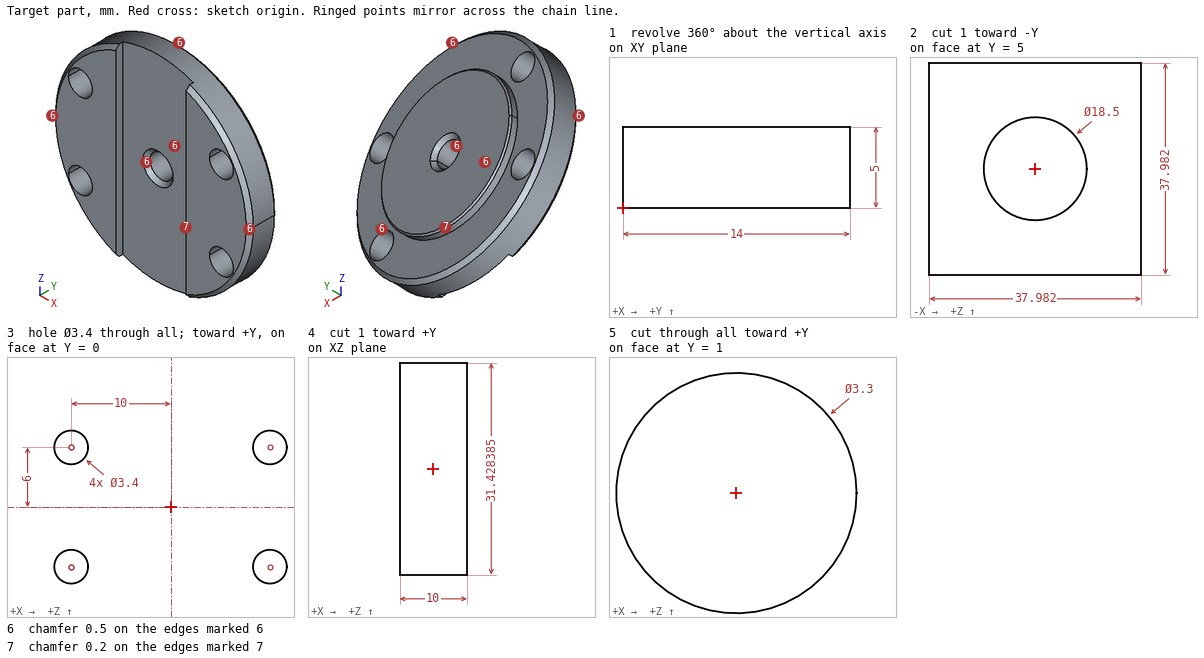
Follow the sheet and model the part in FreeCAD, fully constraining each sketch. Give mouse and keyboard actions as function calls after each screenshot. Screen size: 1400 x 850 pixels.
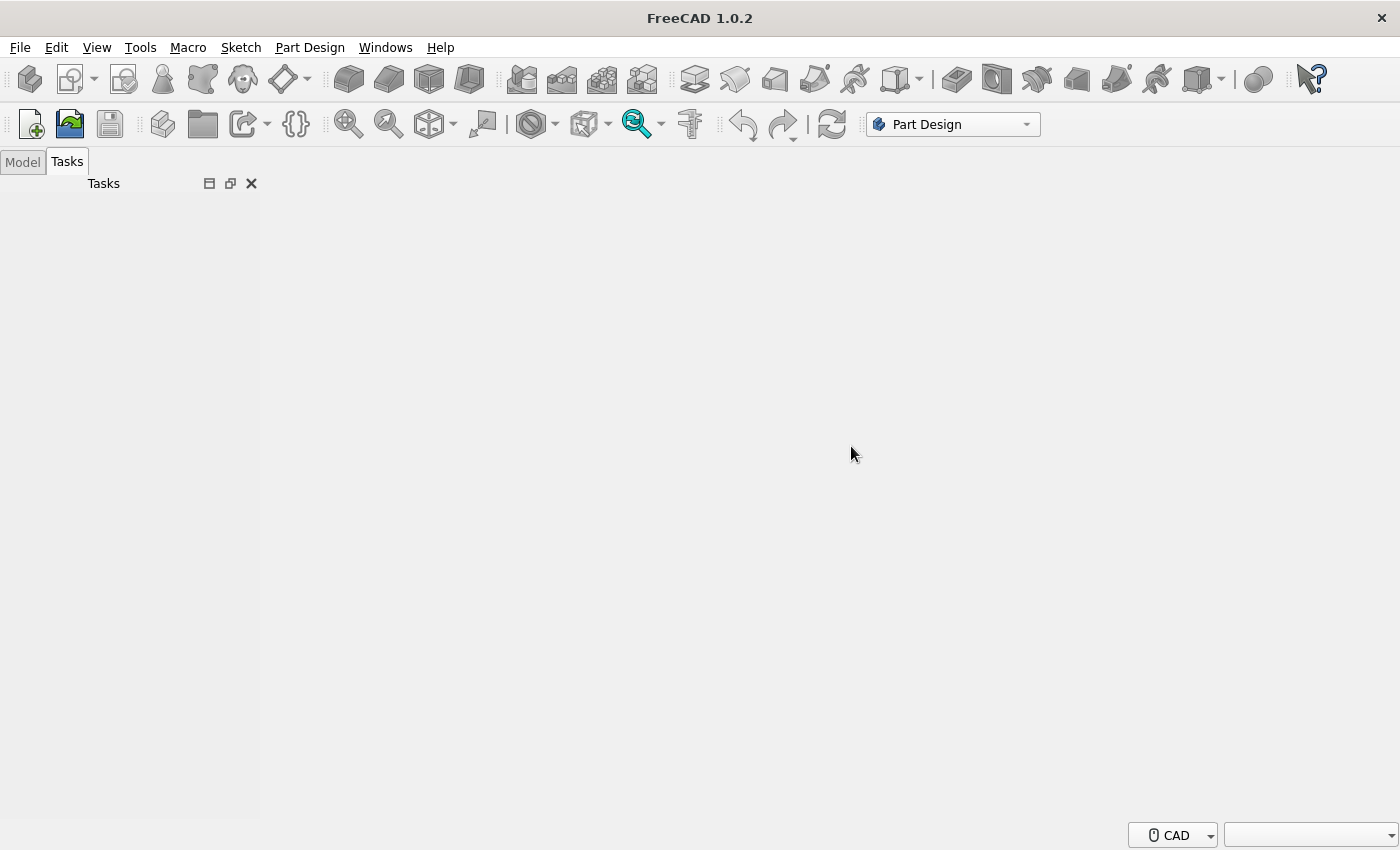
key(ctrl+n)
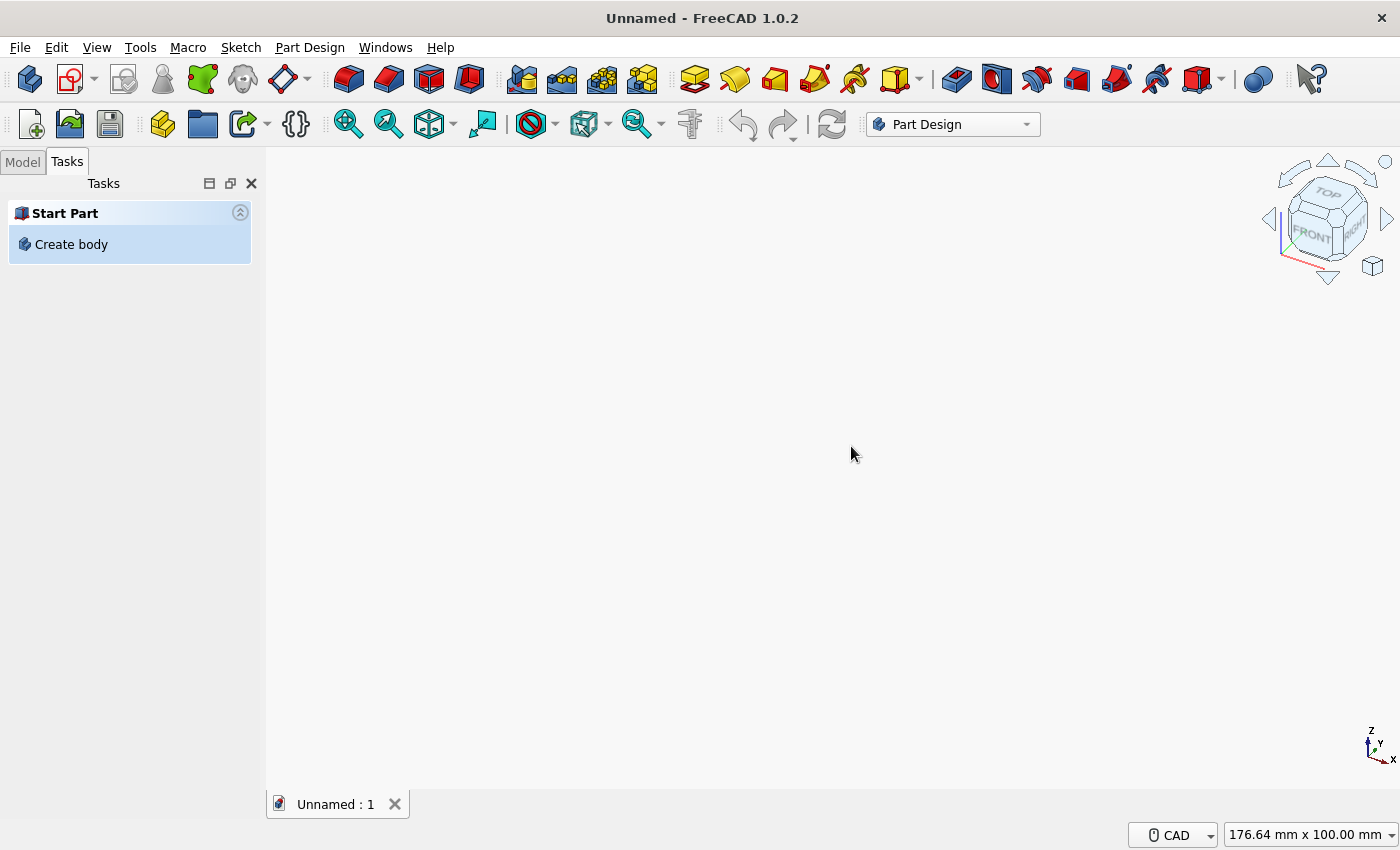
click(70, 80)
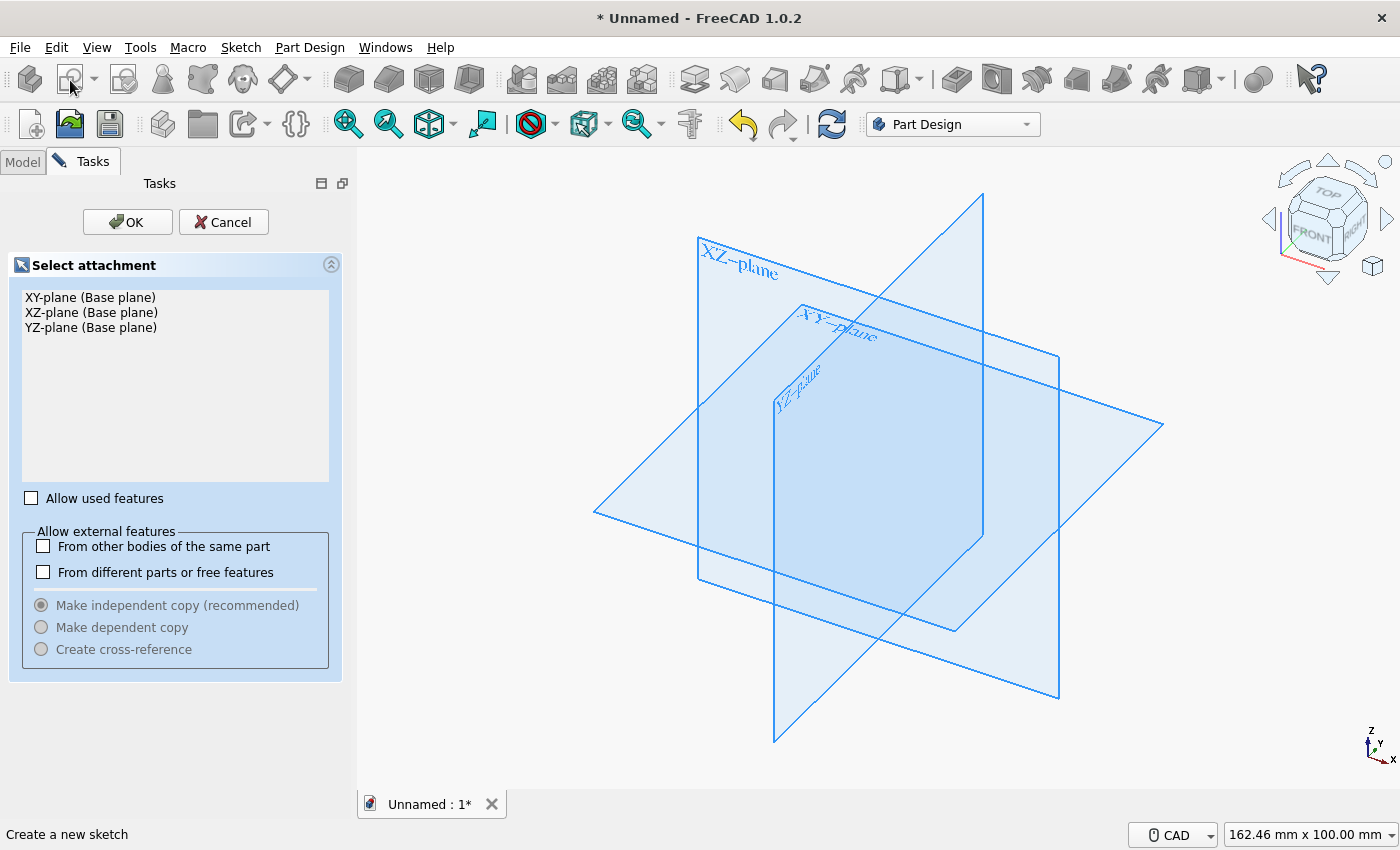
click(82, 298)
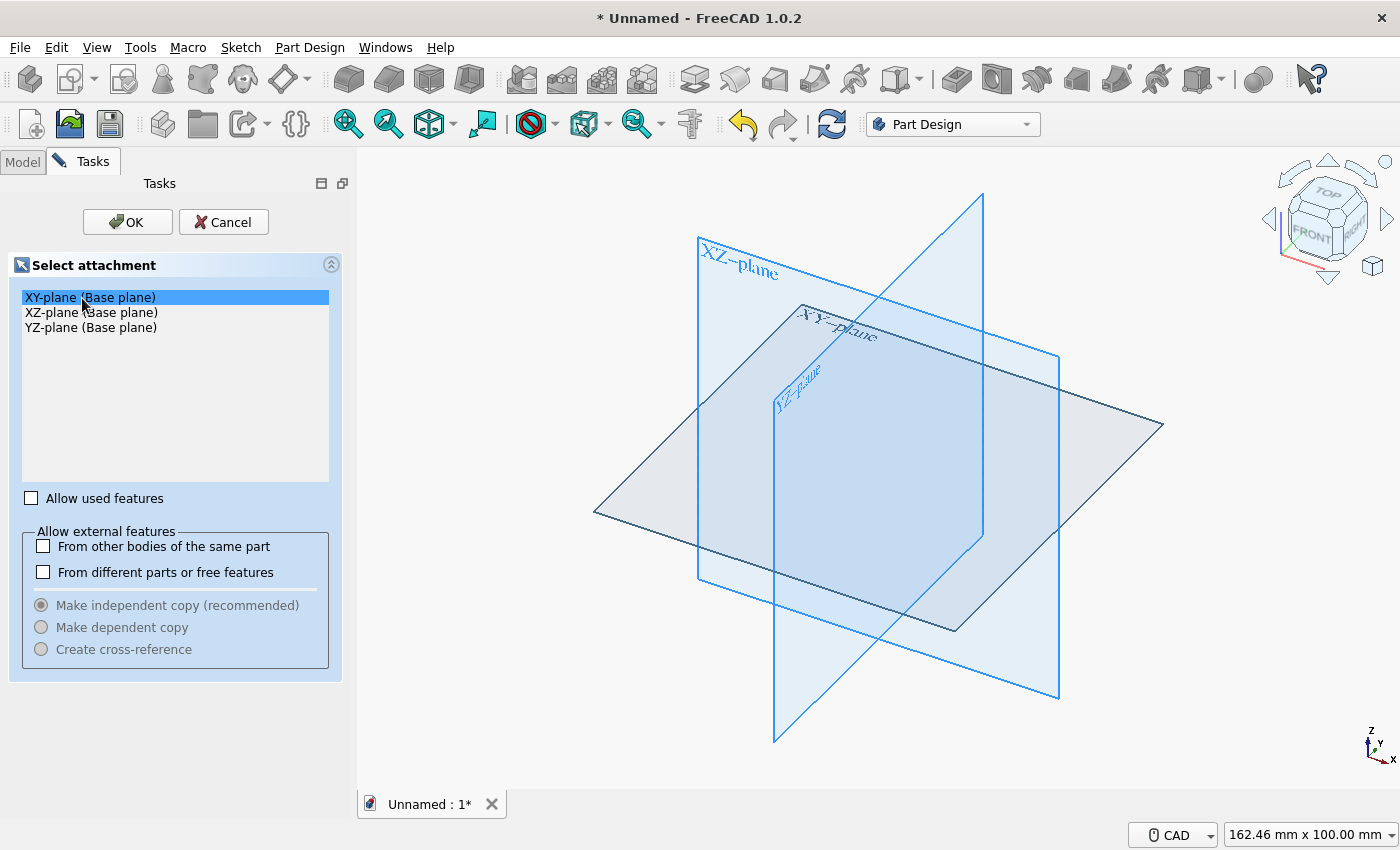
click(128, 222)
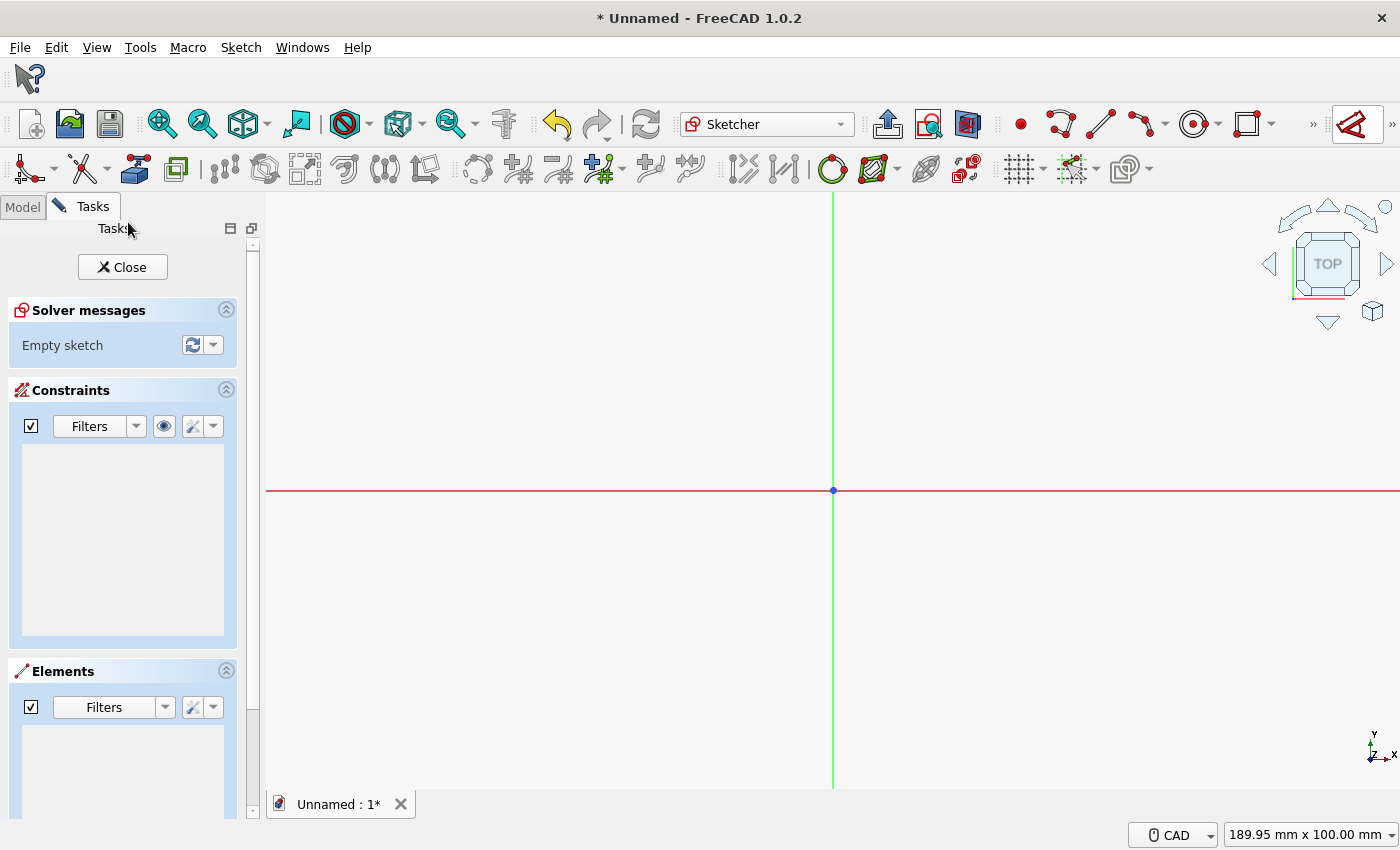
scroll(892, 473, up, 10)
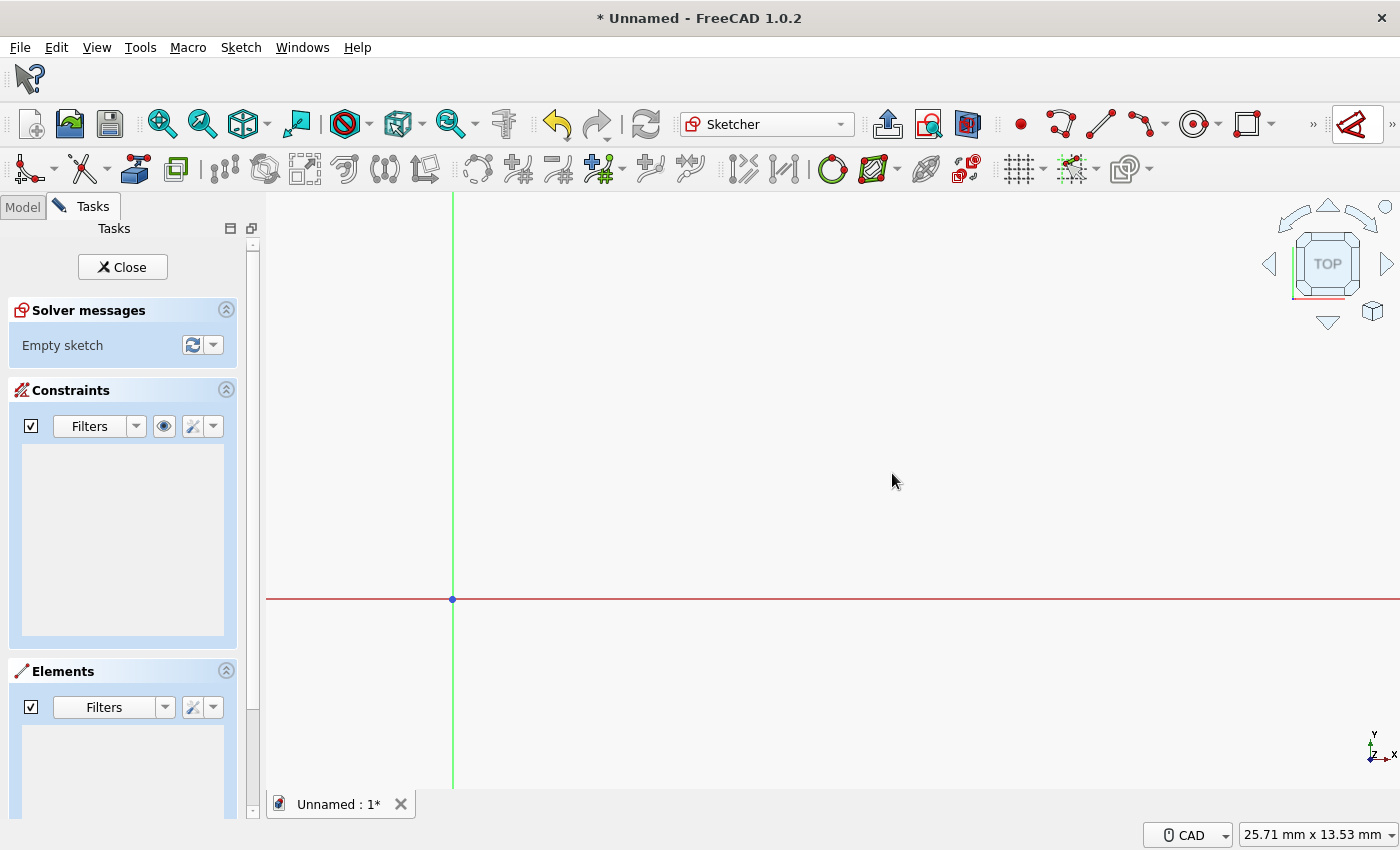
key(g)
key(r)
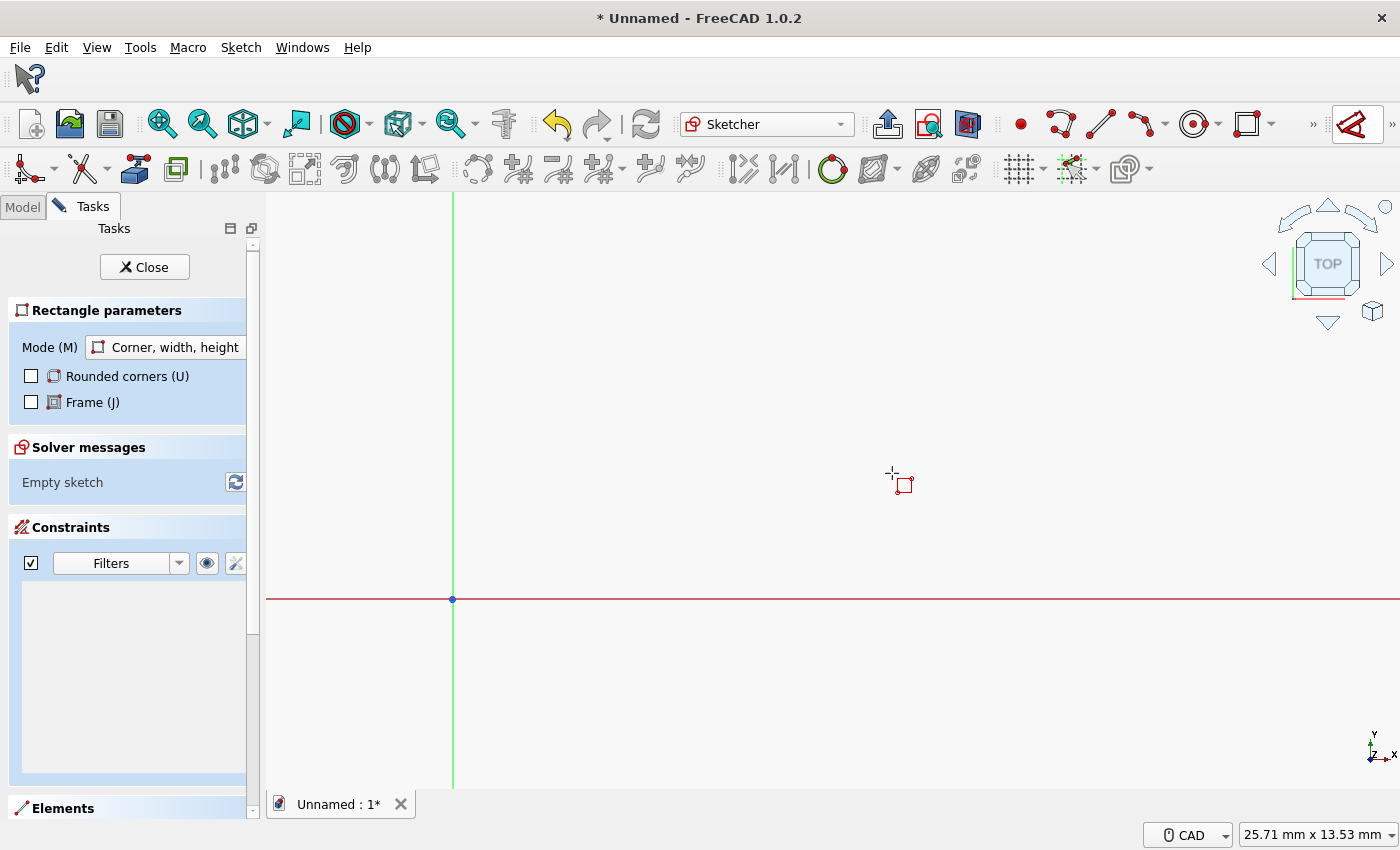
click(453, 599)
move(1070, 379)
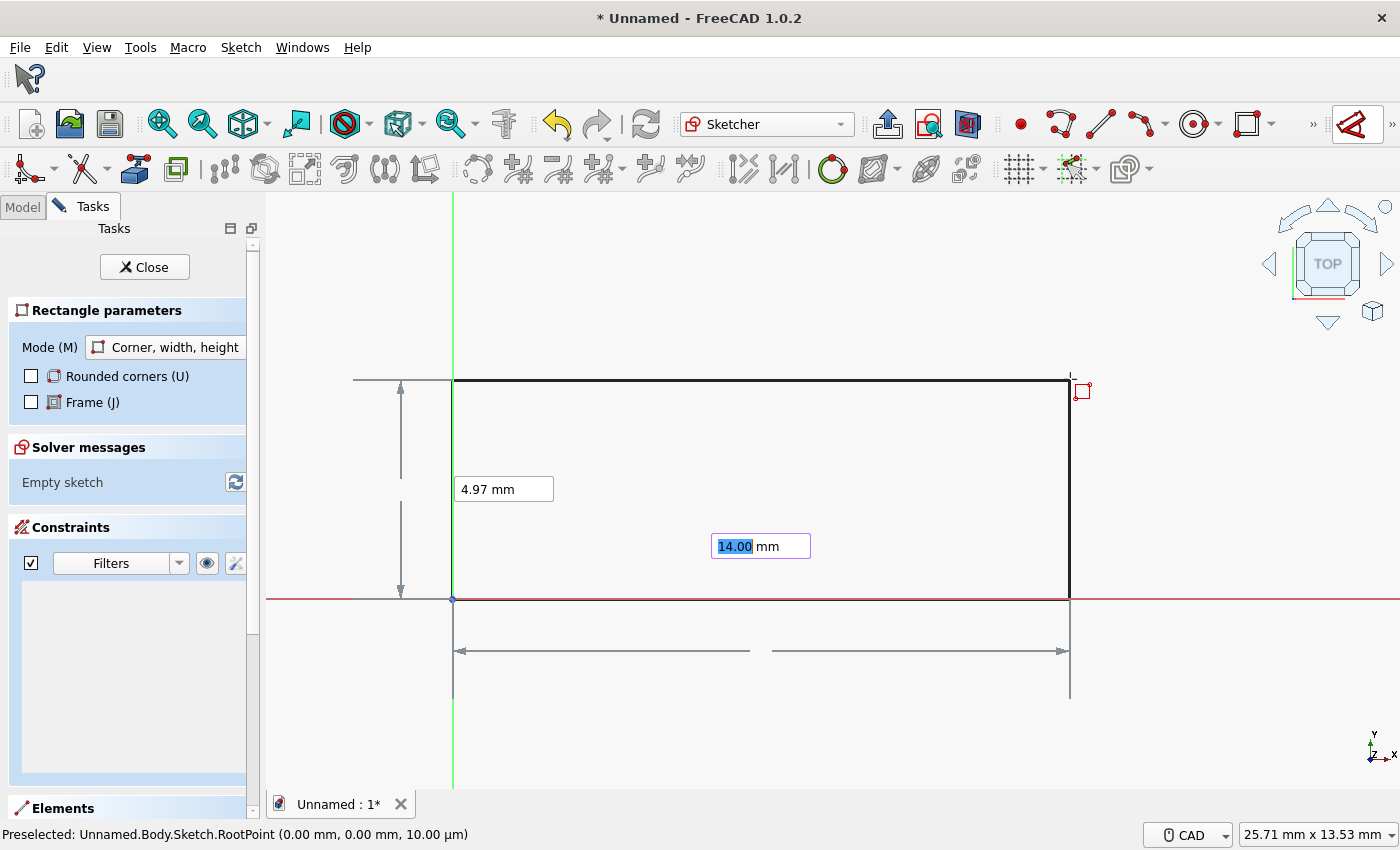
text(14)
key(Tab)
text(5)
key(Return)
key(Escape)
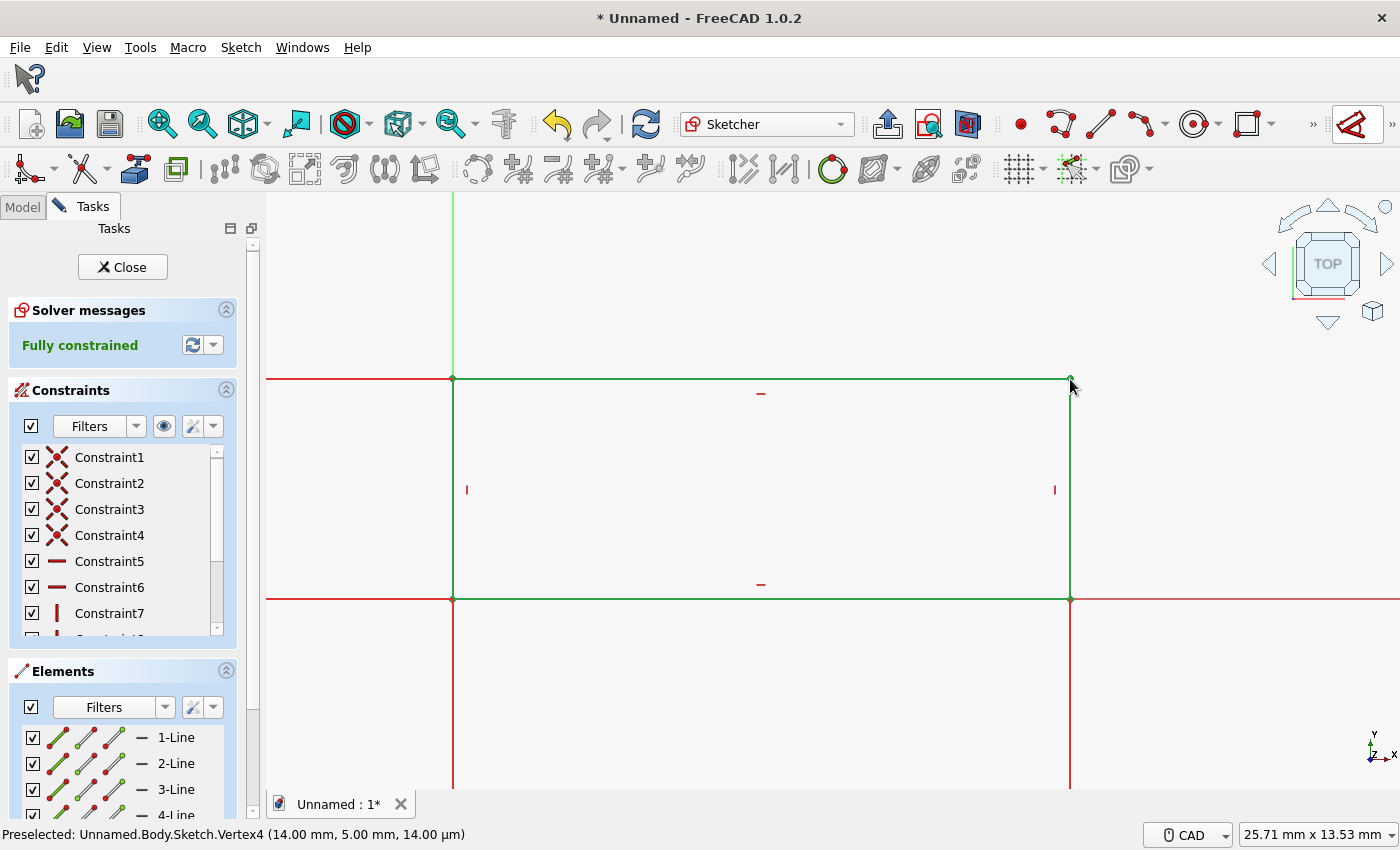
click(123, 267)